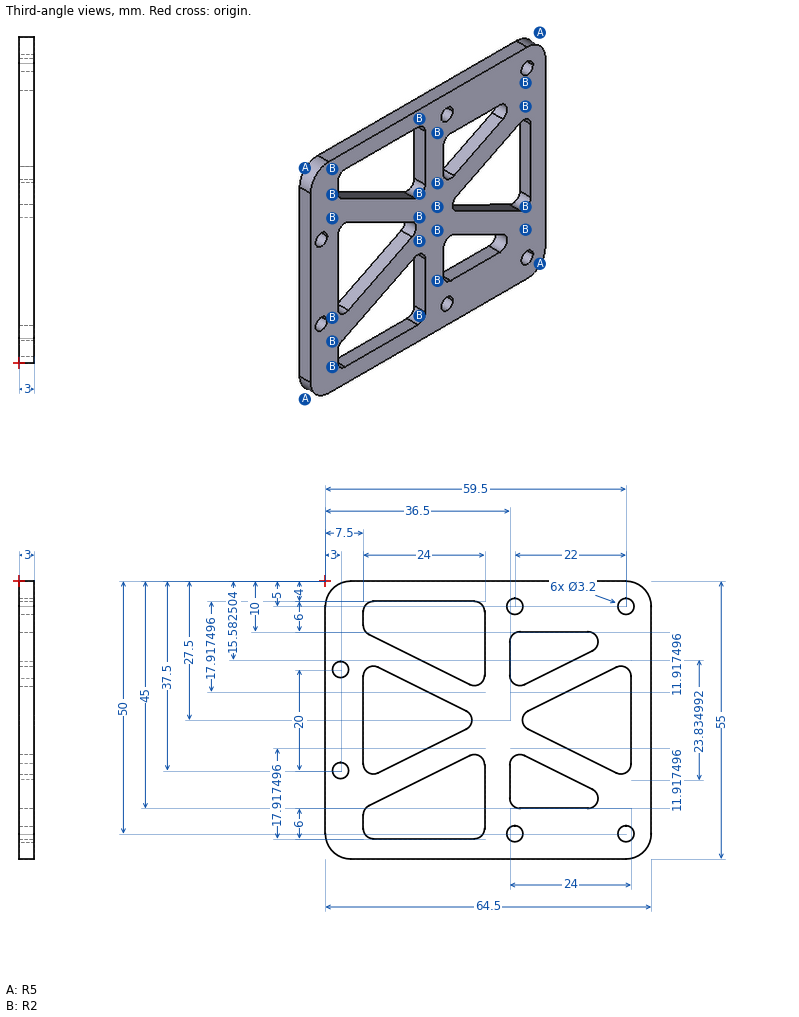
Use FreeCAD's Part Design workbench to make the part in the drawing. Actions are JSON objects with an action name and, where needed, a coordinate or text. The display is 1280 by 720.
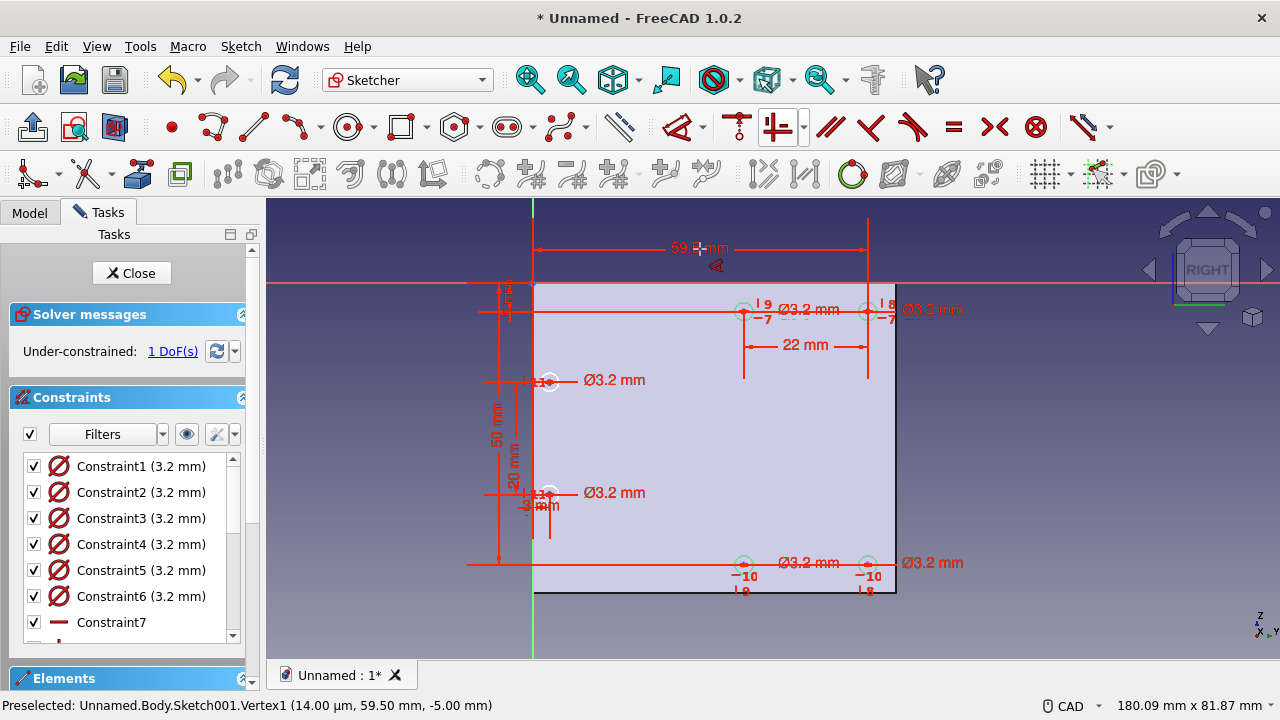
{"action": "left_click", "coordinate": [550, 495]}
{"action": "left_click", "coordinate": [499, 389]}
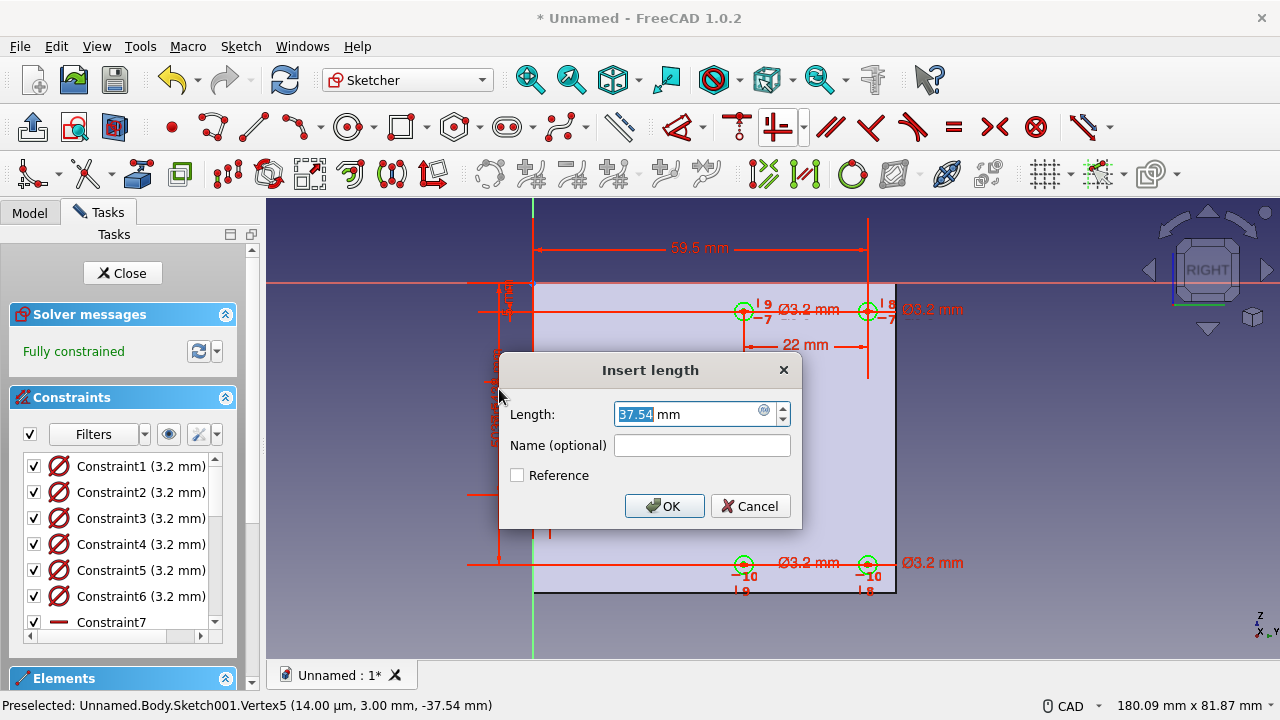
{"action": "type", "text": "37.5"}
{"action": "key", "text": "Return"}
{"action": "key", "text": "Escape"}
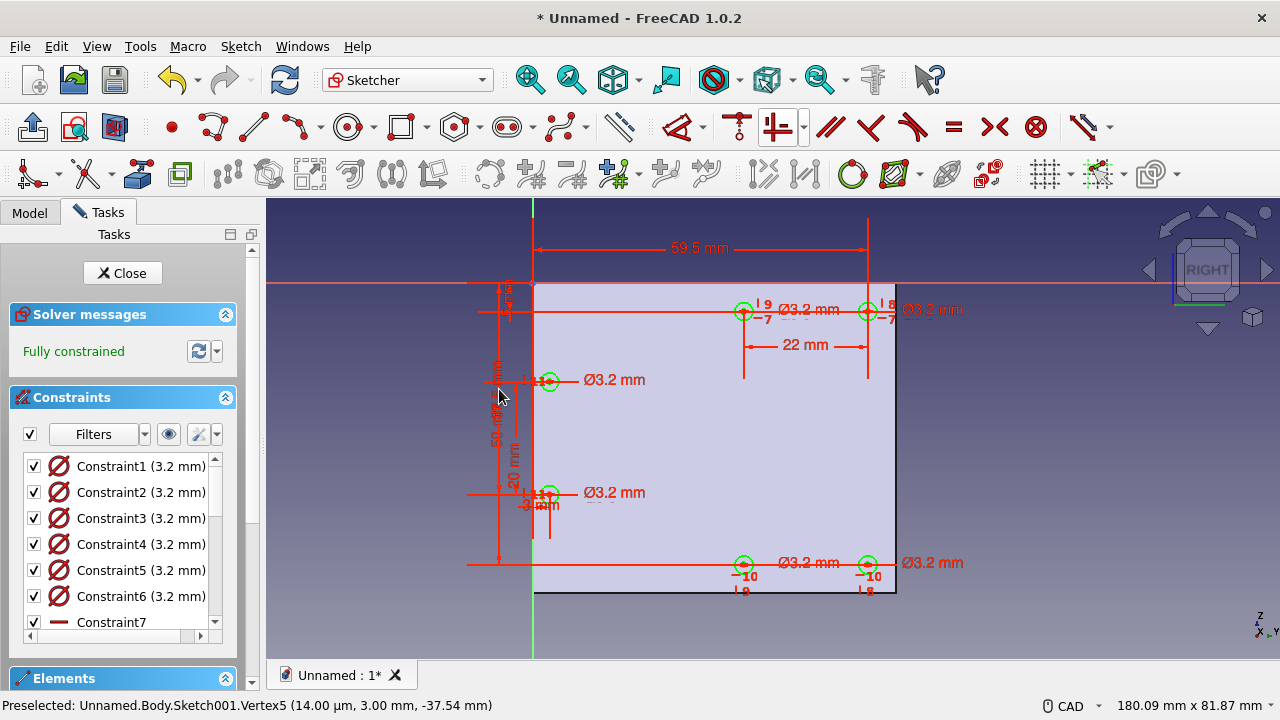
{"action": "left_click", "coordinate": [123, 273]}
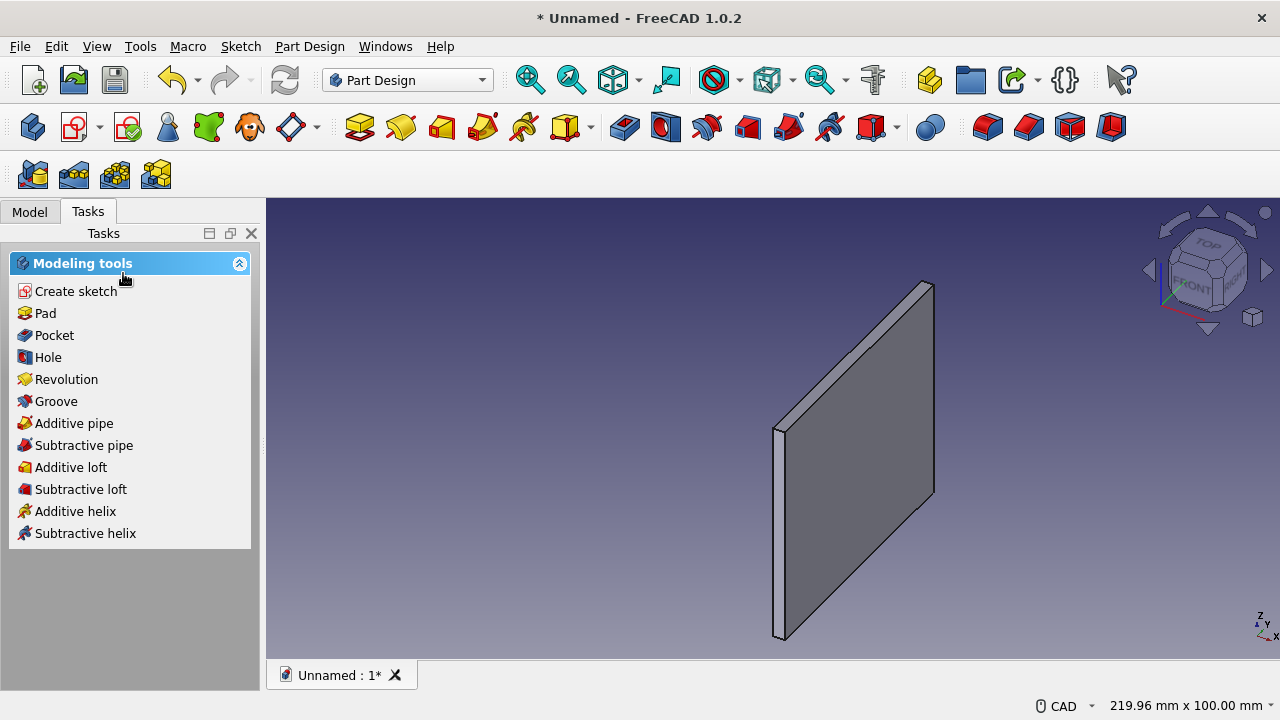
{"action": "left_click", "coordinate": [625, 128]}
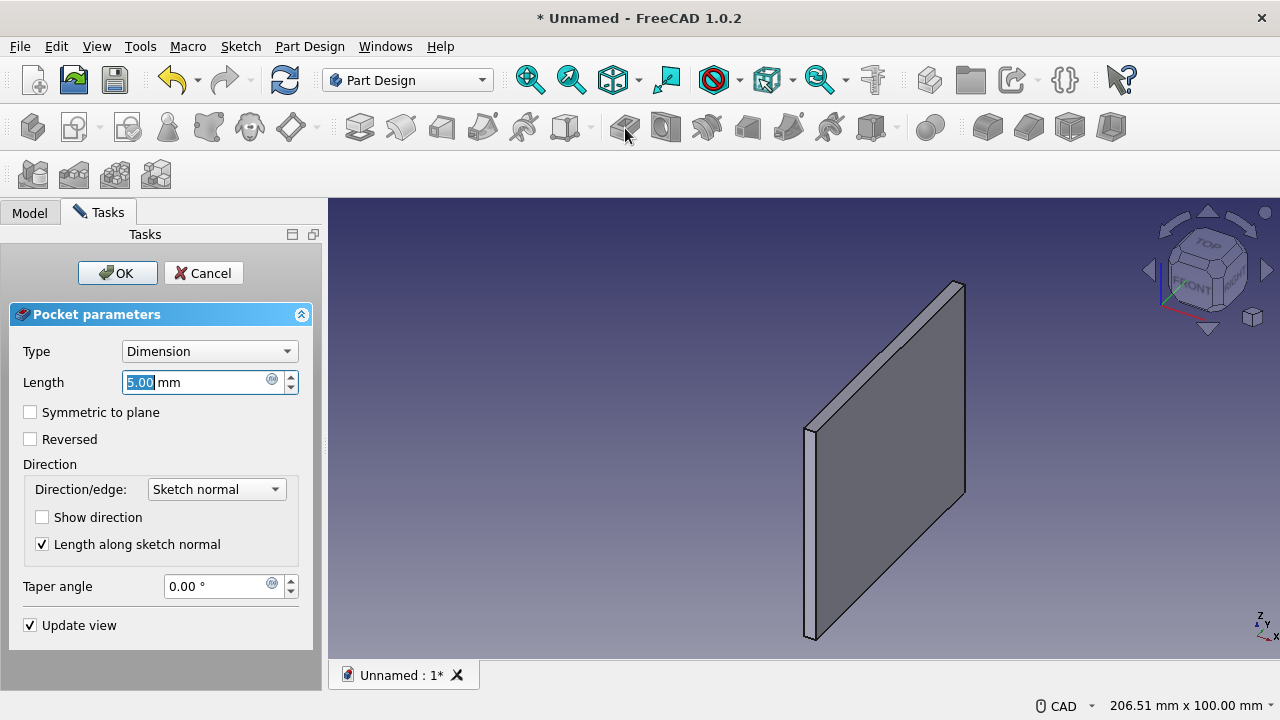
{"action": "type", "text": "3"}
{"action": "key", "text": "Tab"}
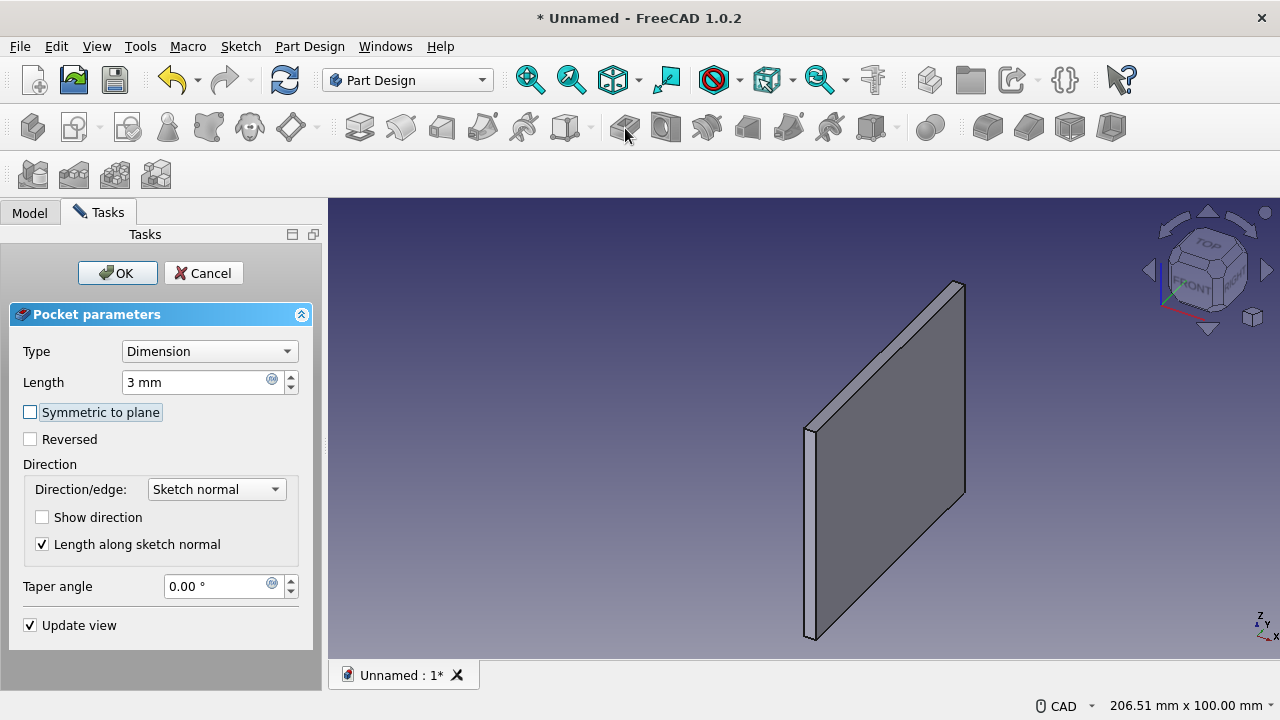
{"action": "left_click", "coordinate": [31, 439]}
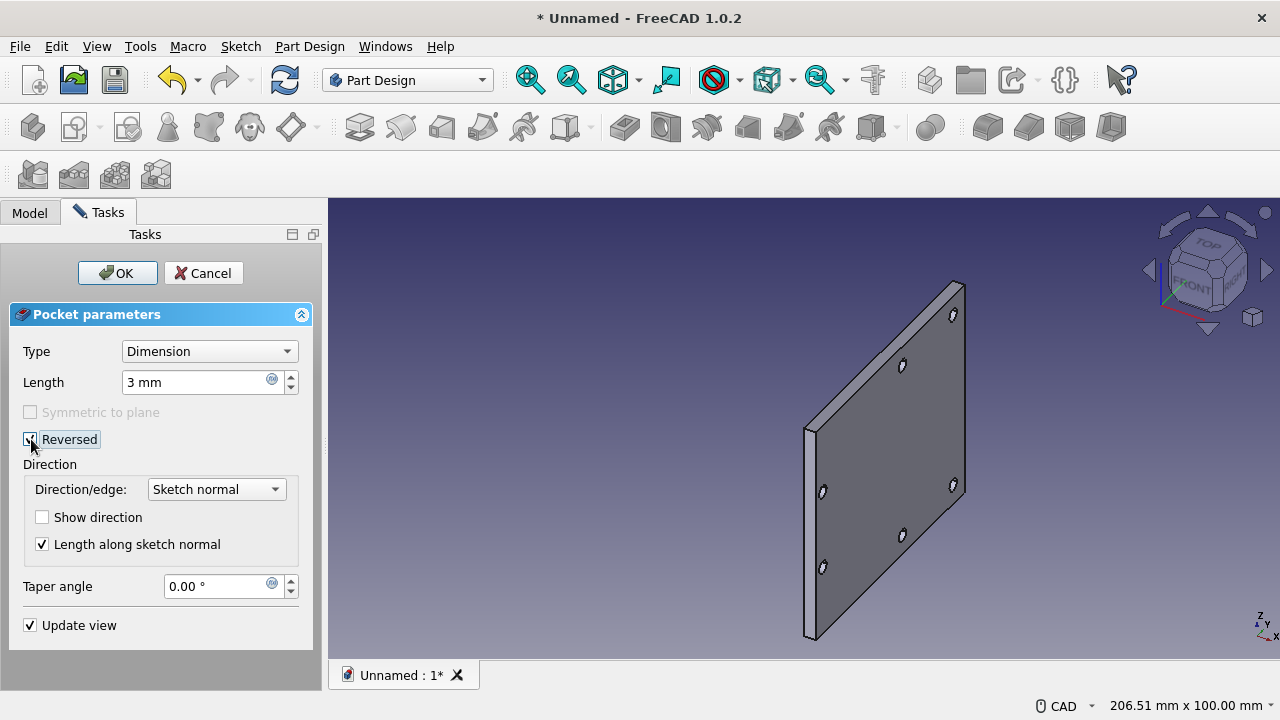
{"action": "left_click", "coordinate": [118, 273]}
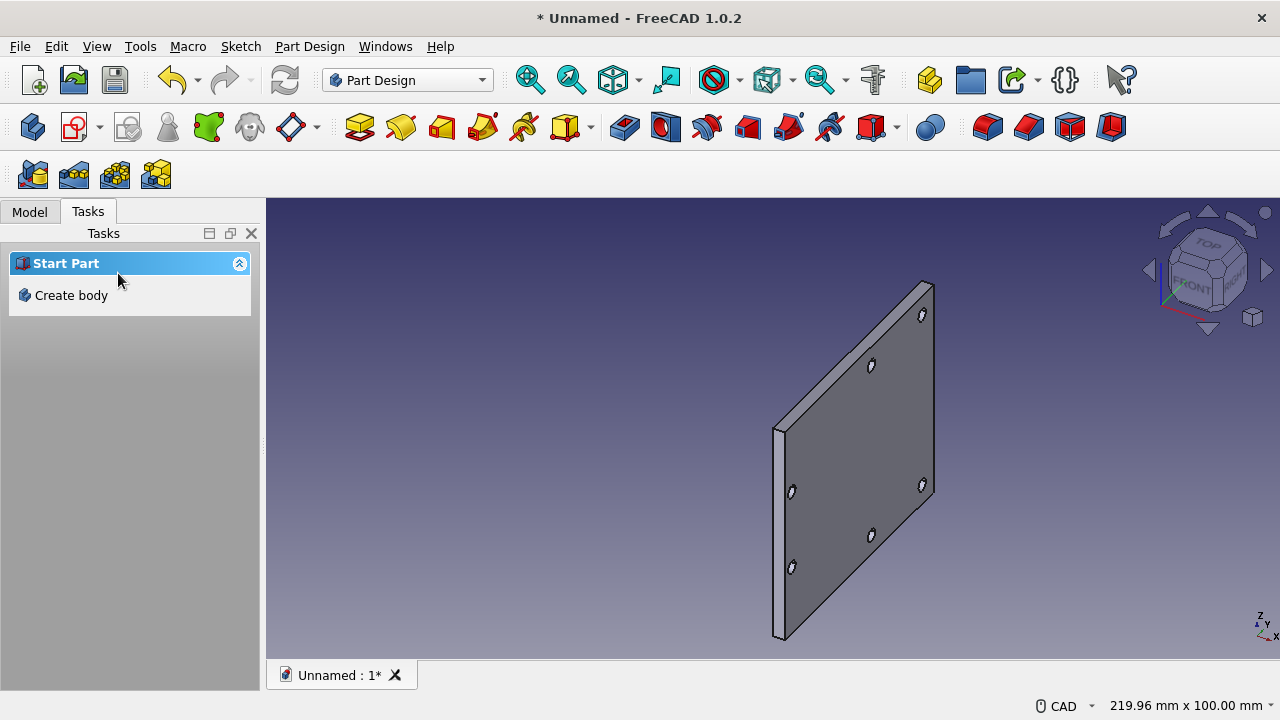
{"action": "left_click", "coordinate": [779, 429]}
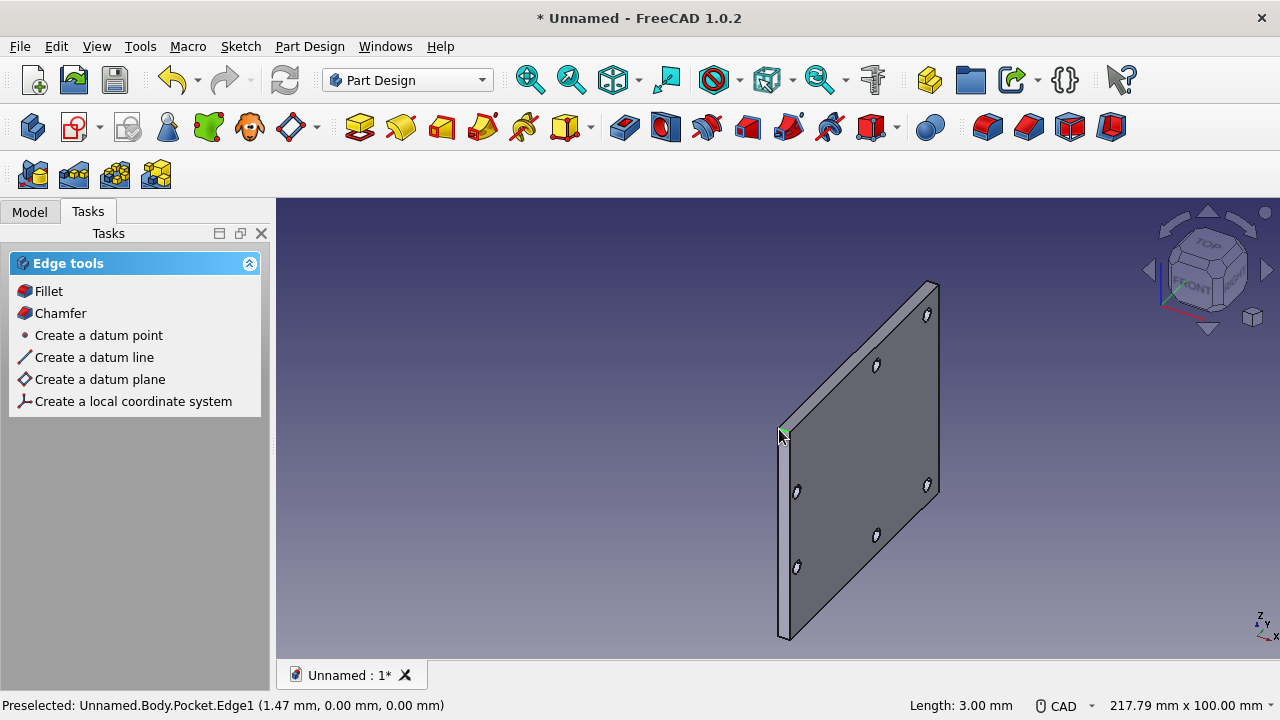
{"action": "scroll", "coordinate": [933, 282], "scroll_direction": "up", "scroll_amount": 6}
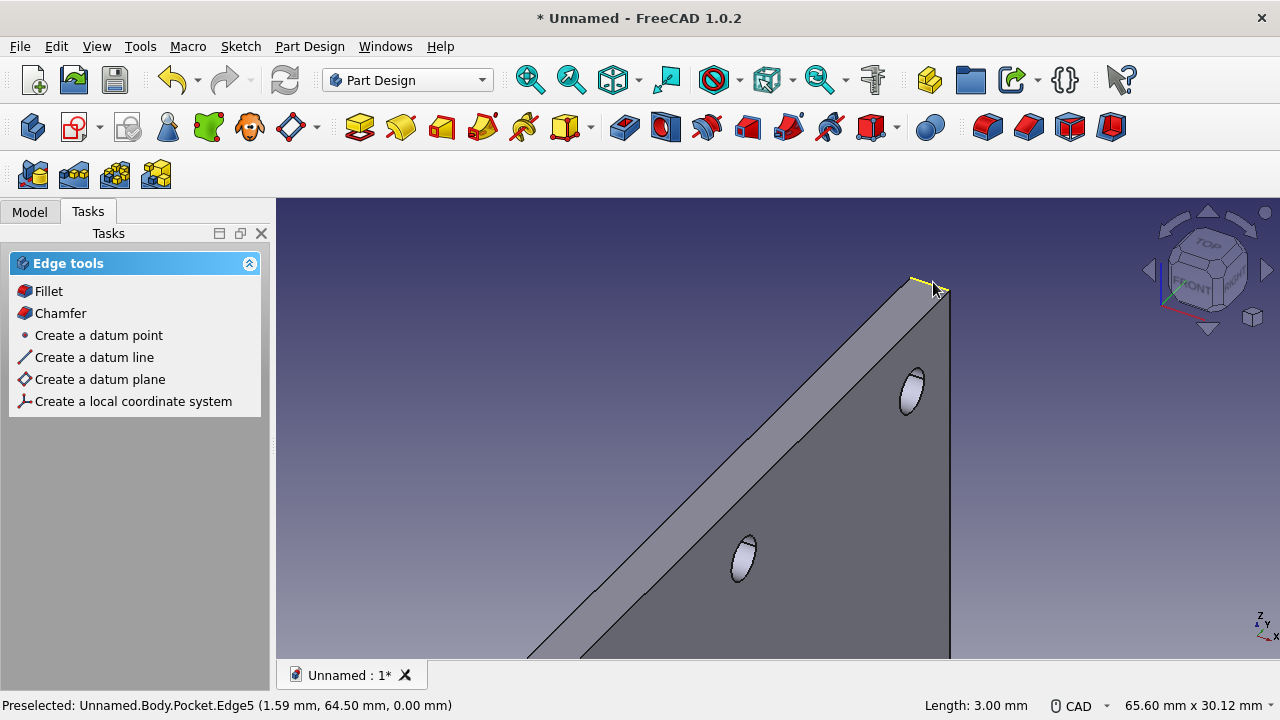
{"action": "left_click", "coordinate": [531, 80]}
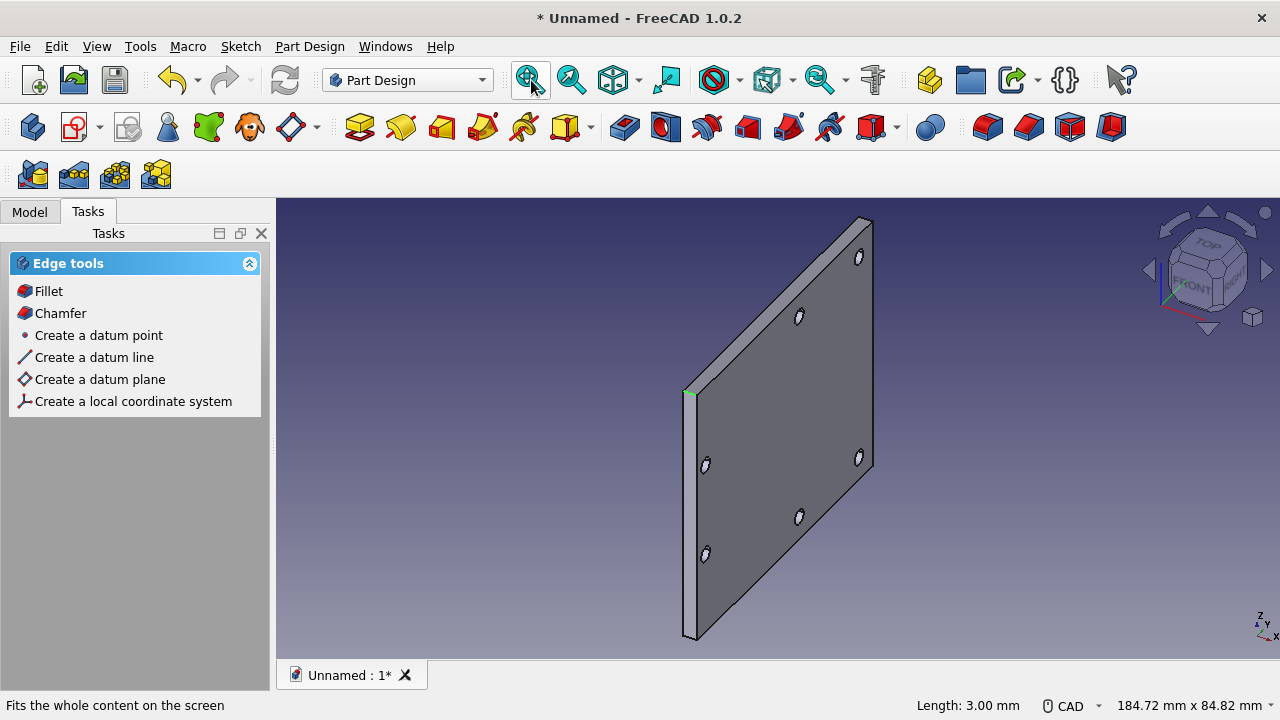
{"action": "key", "text": "0"}